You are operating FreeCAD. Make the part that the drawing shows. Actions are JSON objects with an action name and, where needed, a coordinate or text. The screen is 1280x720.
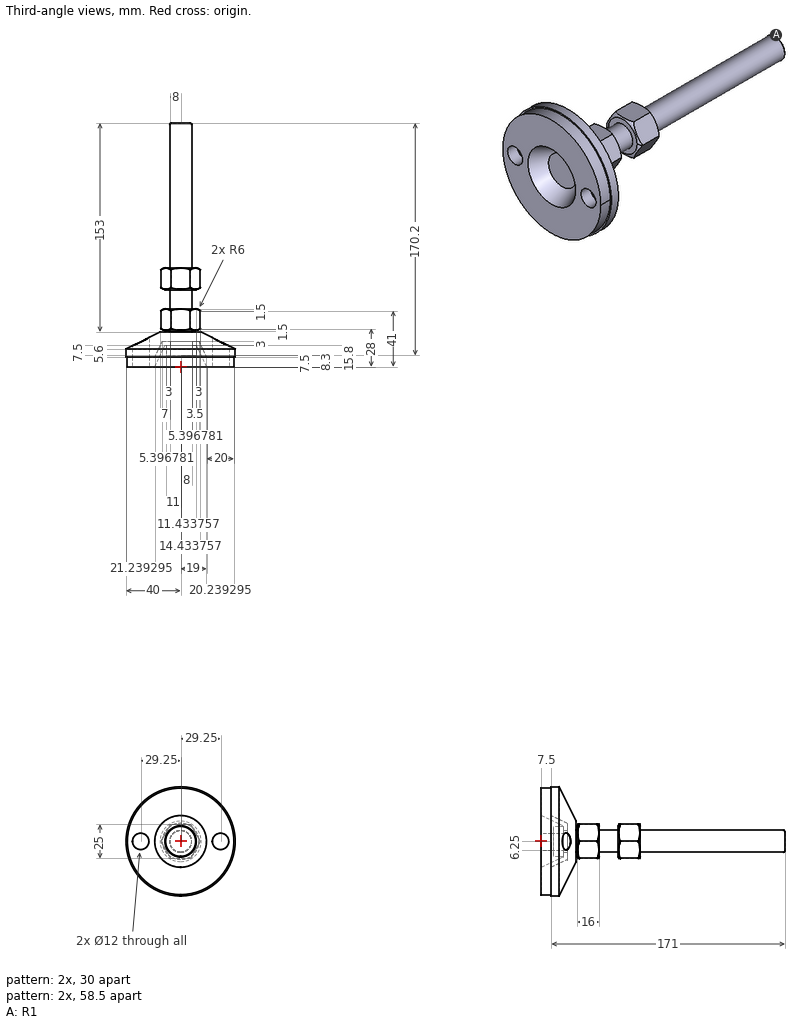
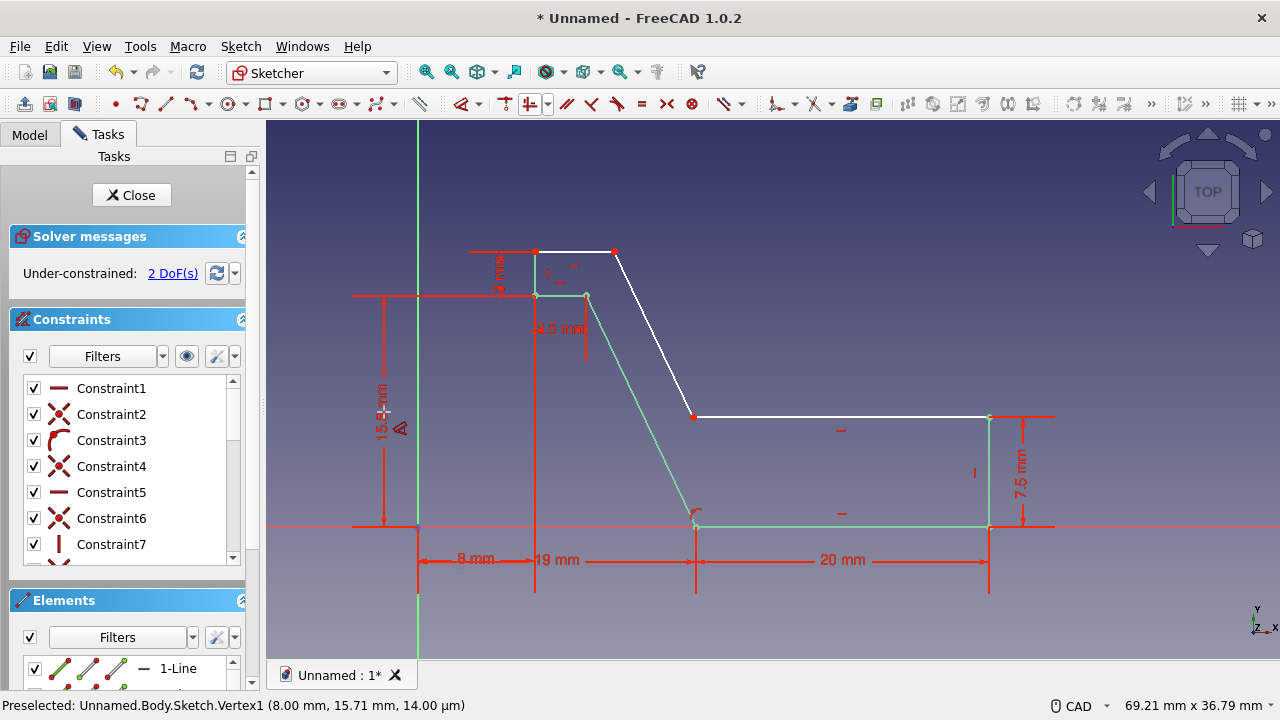
{"action": "left_click", "coordinate": [590, 252]}
{"action": "left_click", "coordinate": [575, 218]}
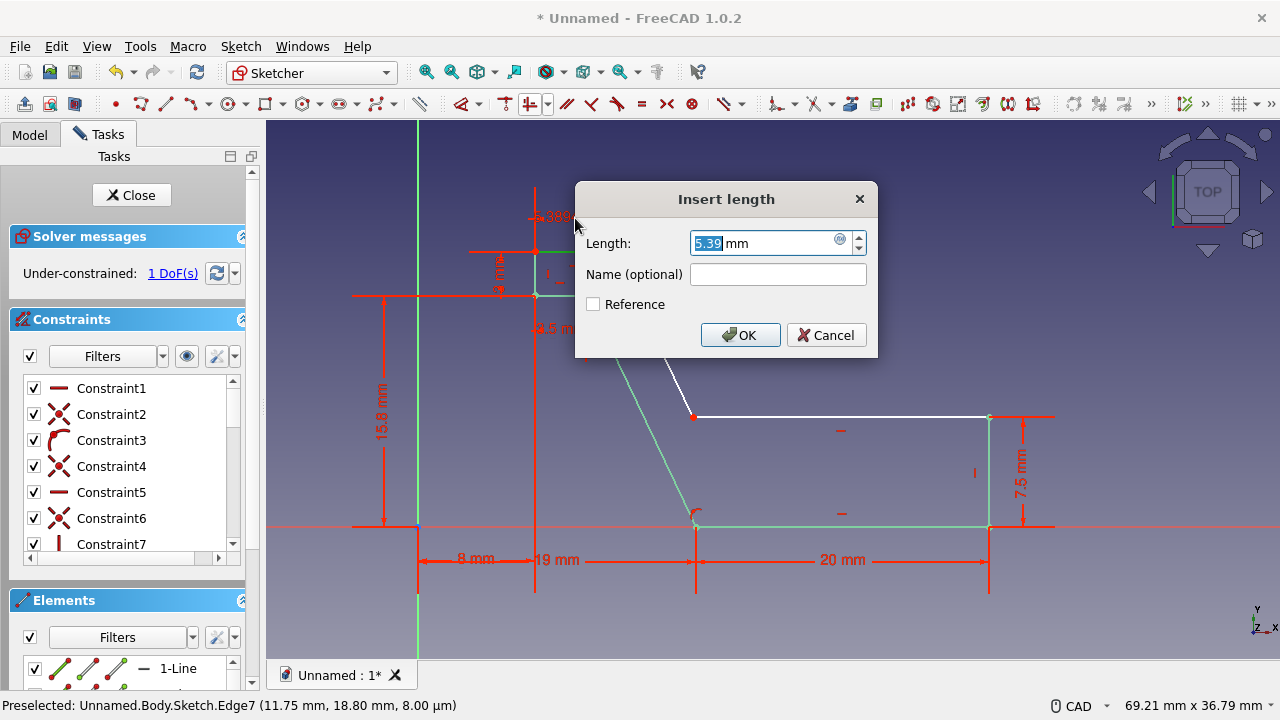
{"action": "type", "text": "5.396781"}
{"action": "key", "text": "Return"}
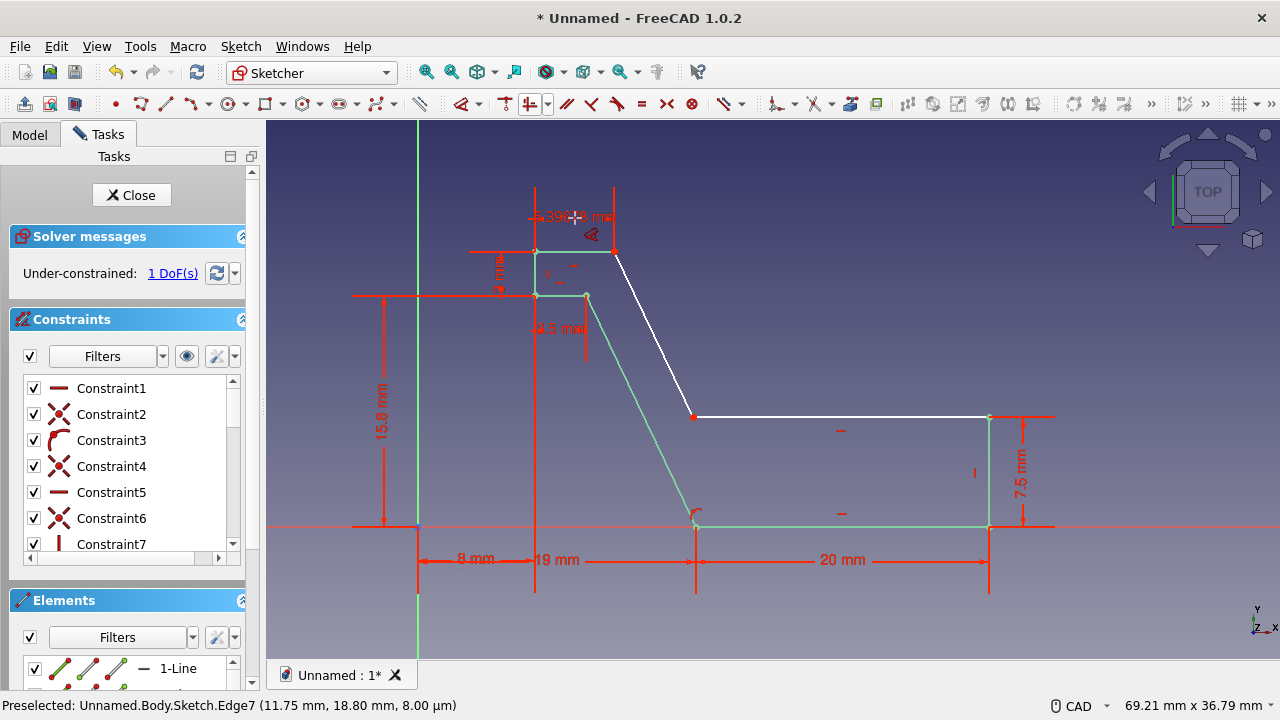
{"action": "left_click", "coordinate": [900, 417]}
{"action": "left_click", "coordinate": [841, 451]}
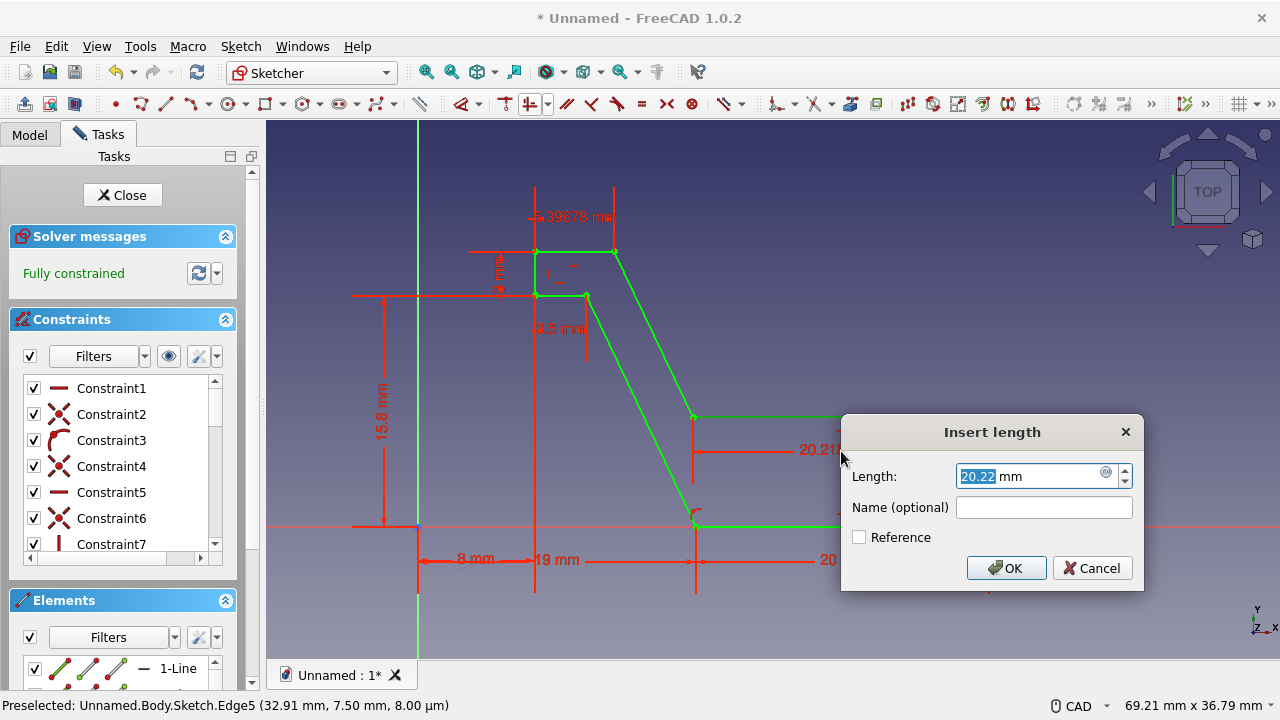
{"action": "type", "text": "20.239295"}
{"action": "key", "text": "Return"}
{"action": "key", "text": "Escape"}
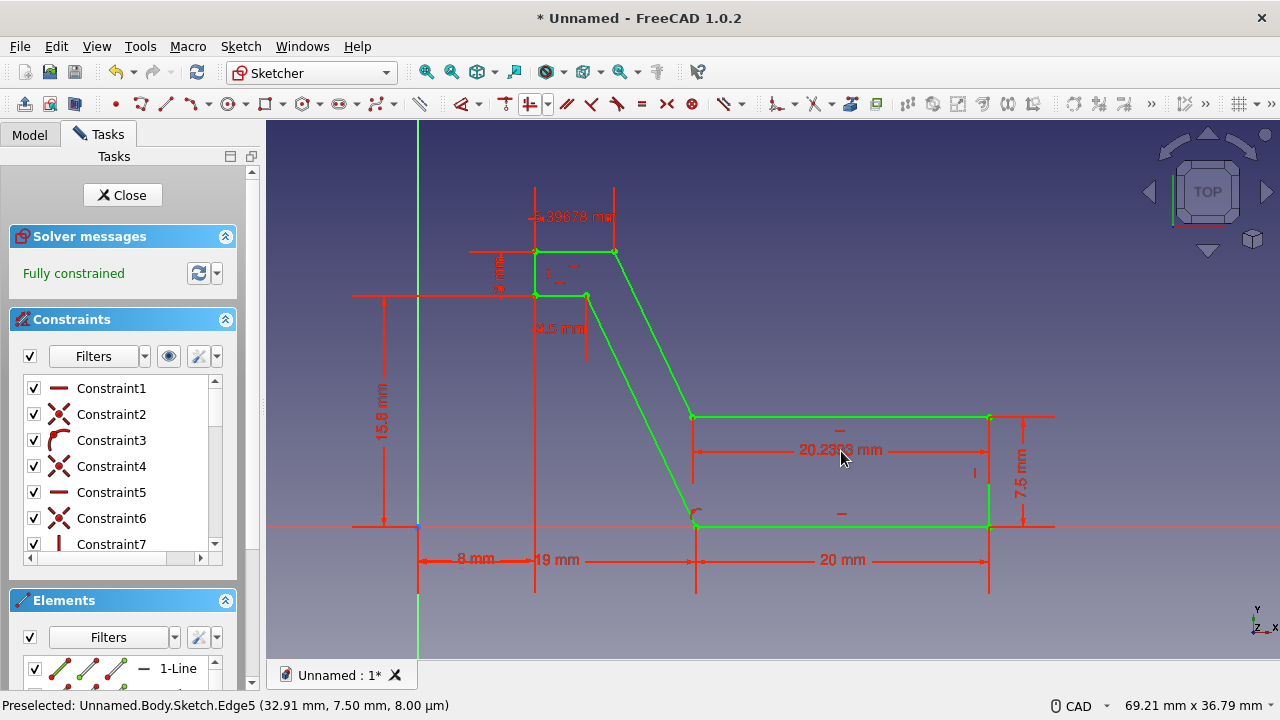
{"action": "left_click", "coordinate": [123, 195]}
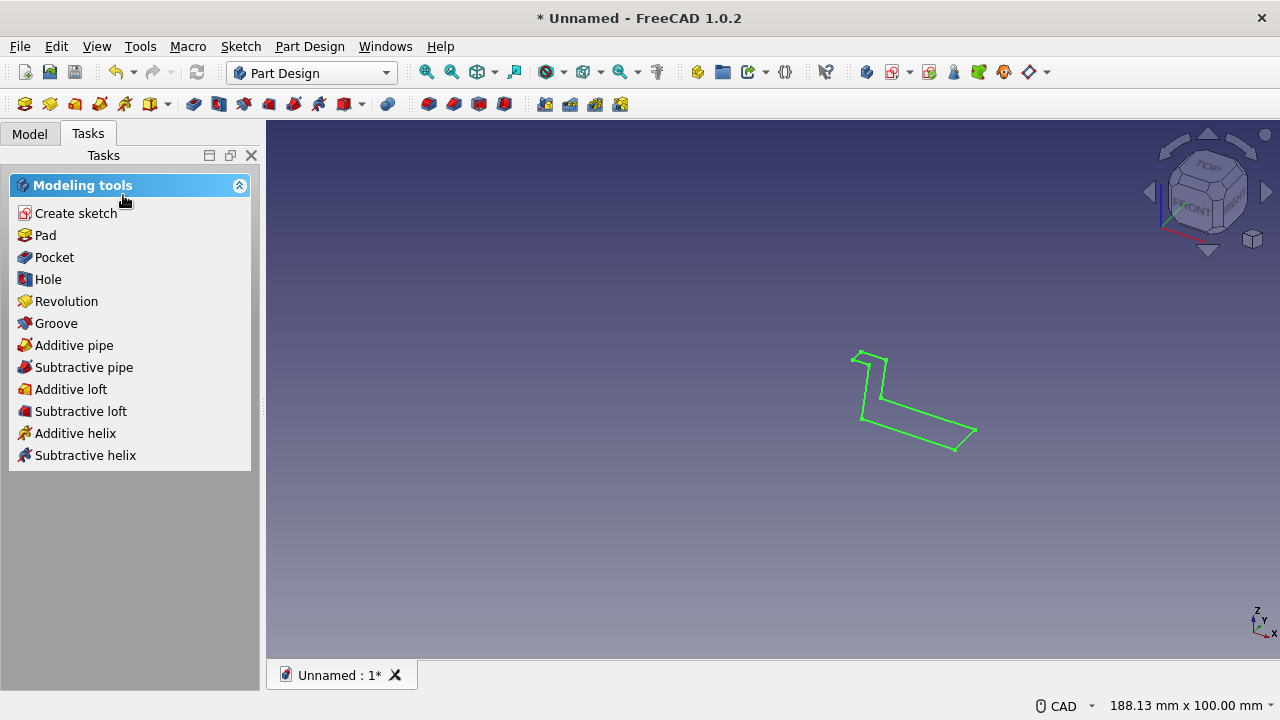
{"action": "left_click", "coordinate": [50, 104]}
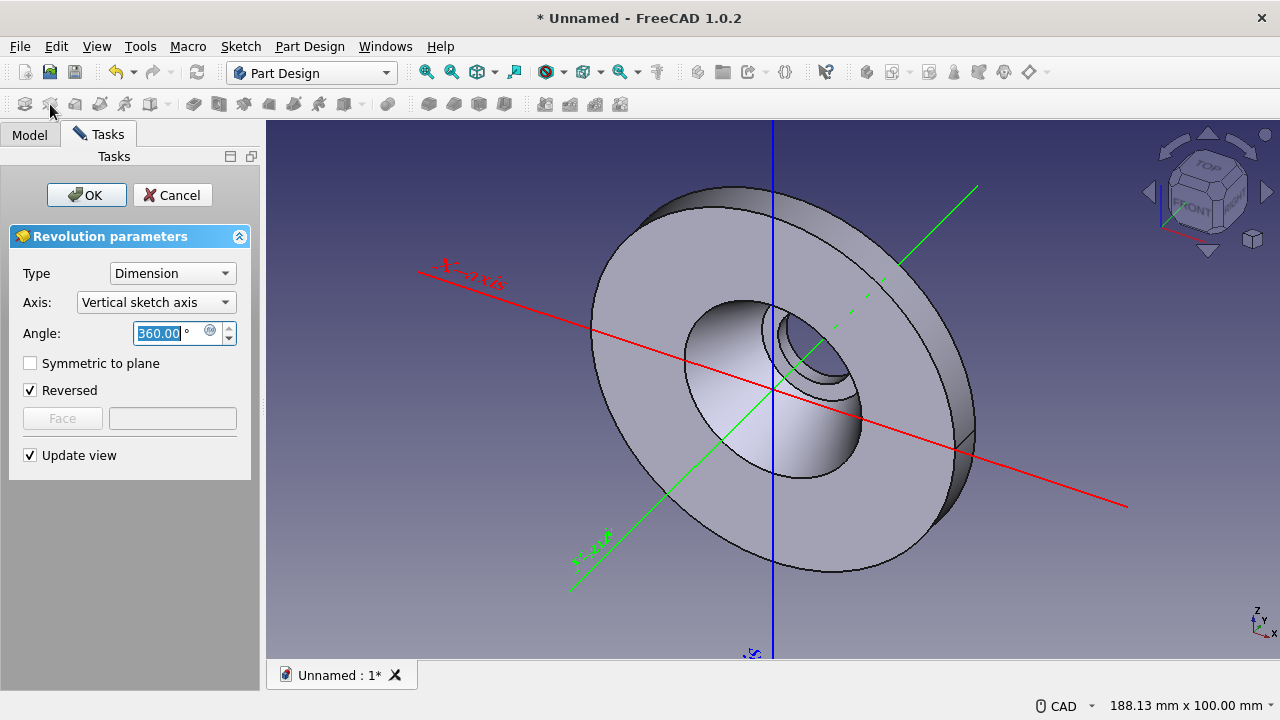
{"action": "left_click", "coordinate": [87, 195]}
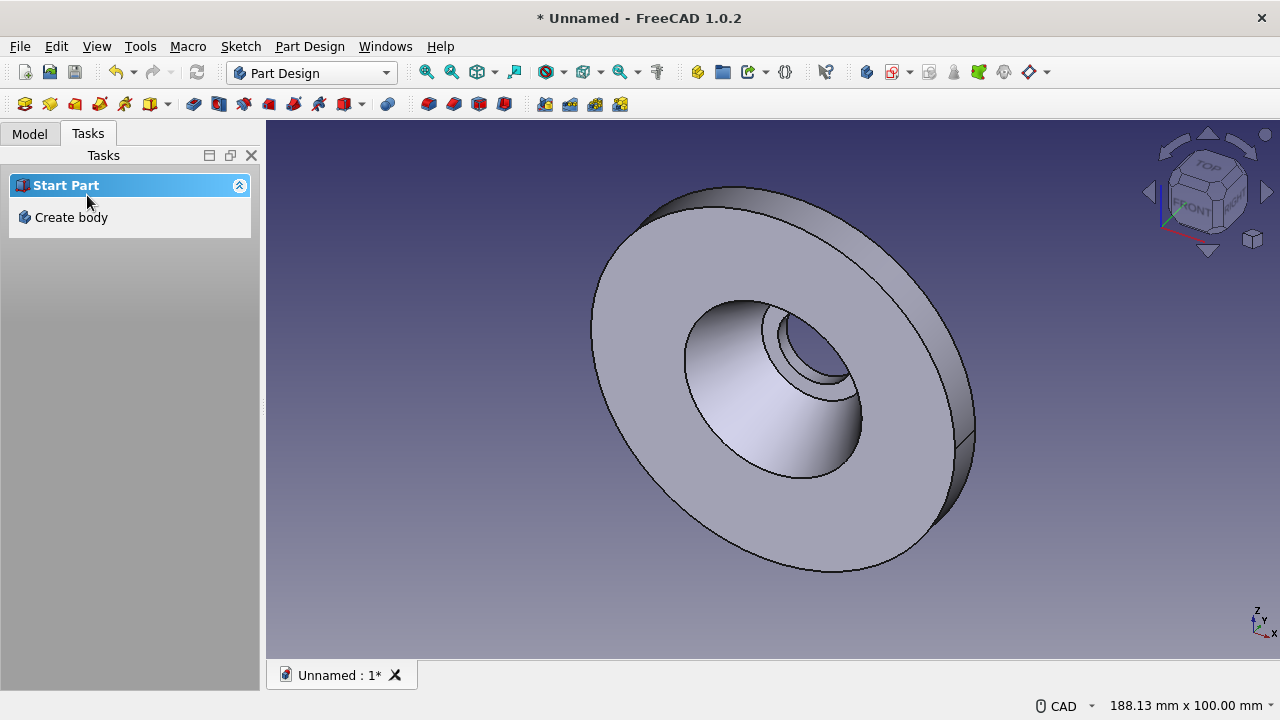
{"action": "left_click", "coordinate": [427, 72]}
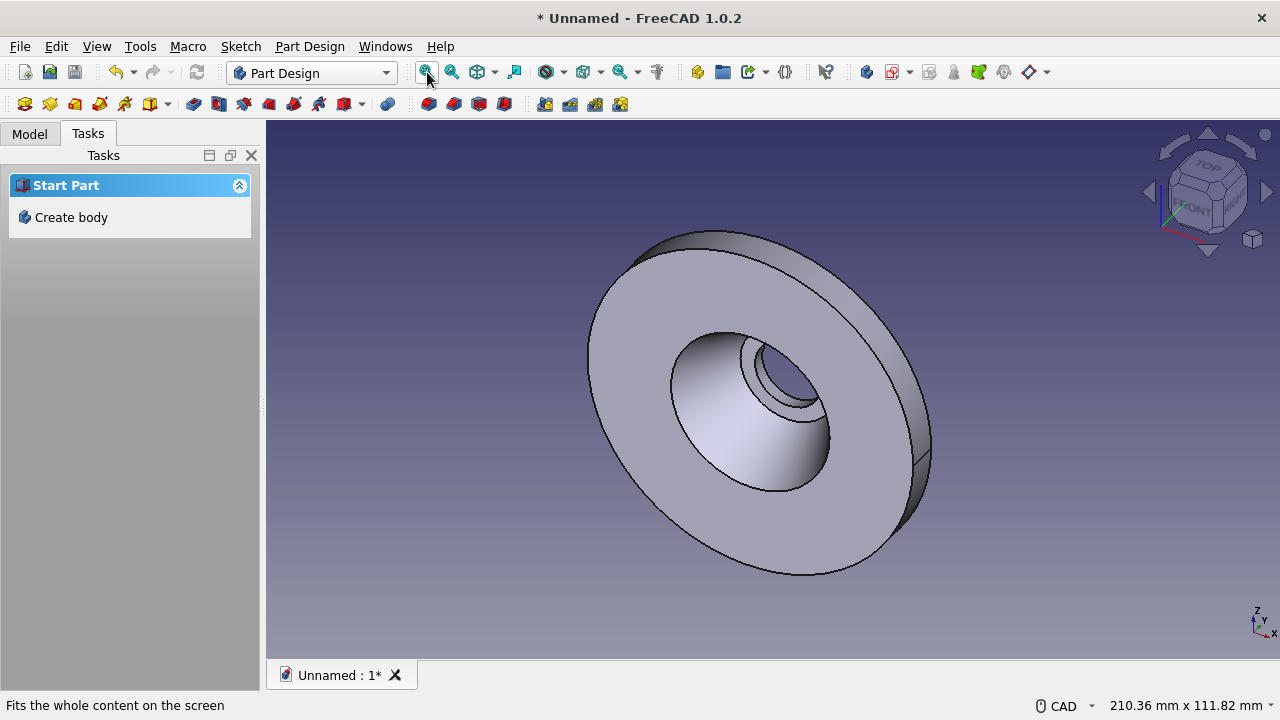
{"action": "key", "text": "4"}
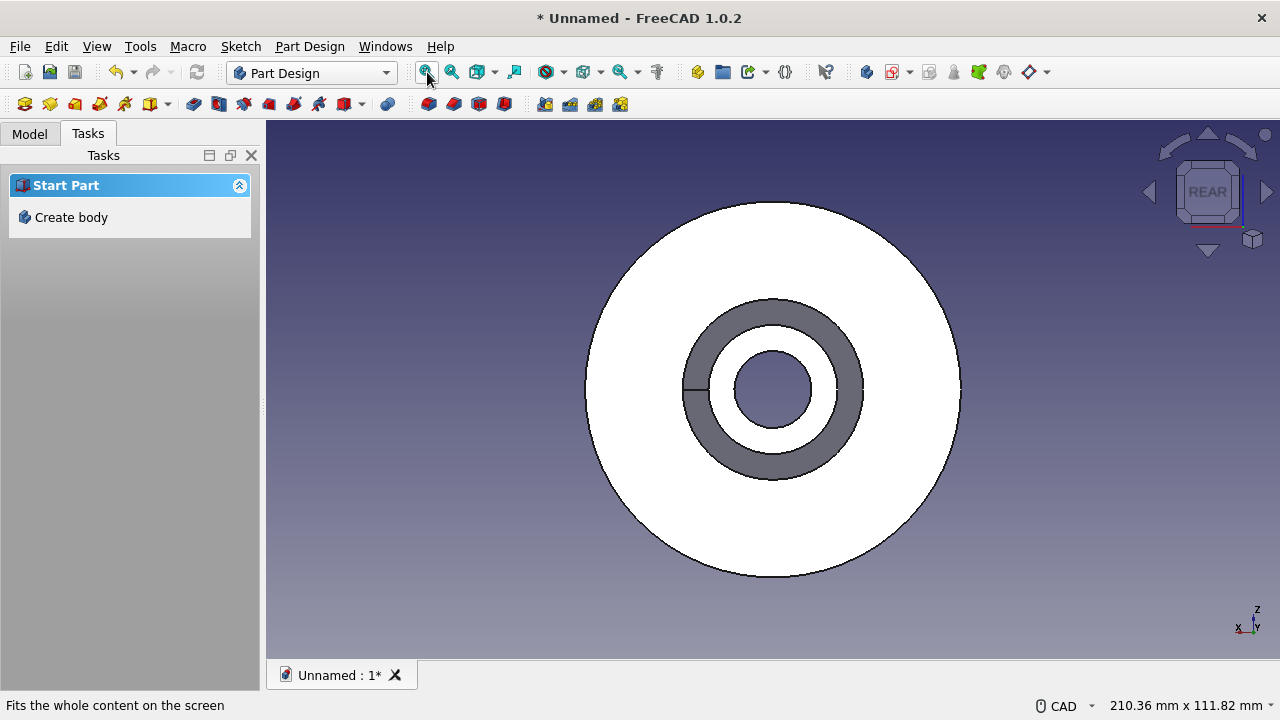
{"action": "left_click", "coordinate": [880, 496]}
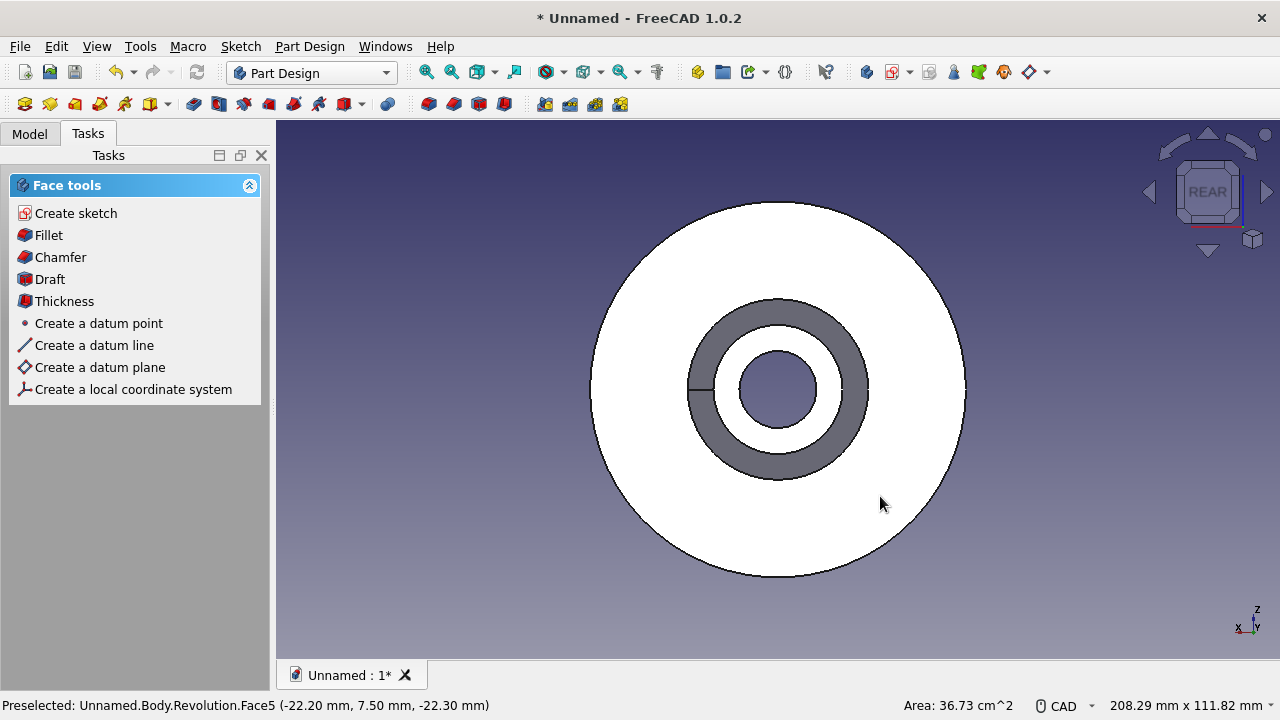
{"action": "left_click", "coordinate": [892, 72]}